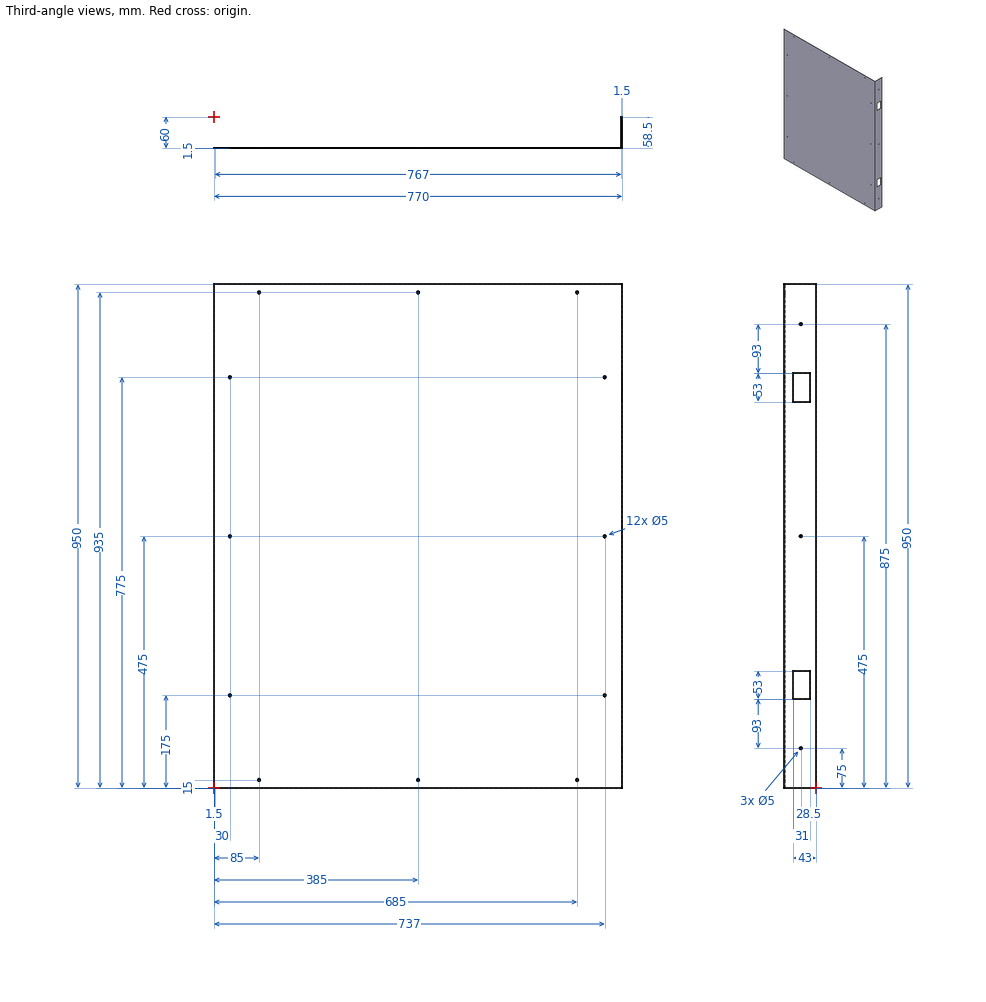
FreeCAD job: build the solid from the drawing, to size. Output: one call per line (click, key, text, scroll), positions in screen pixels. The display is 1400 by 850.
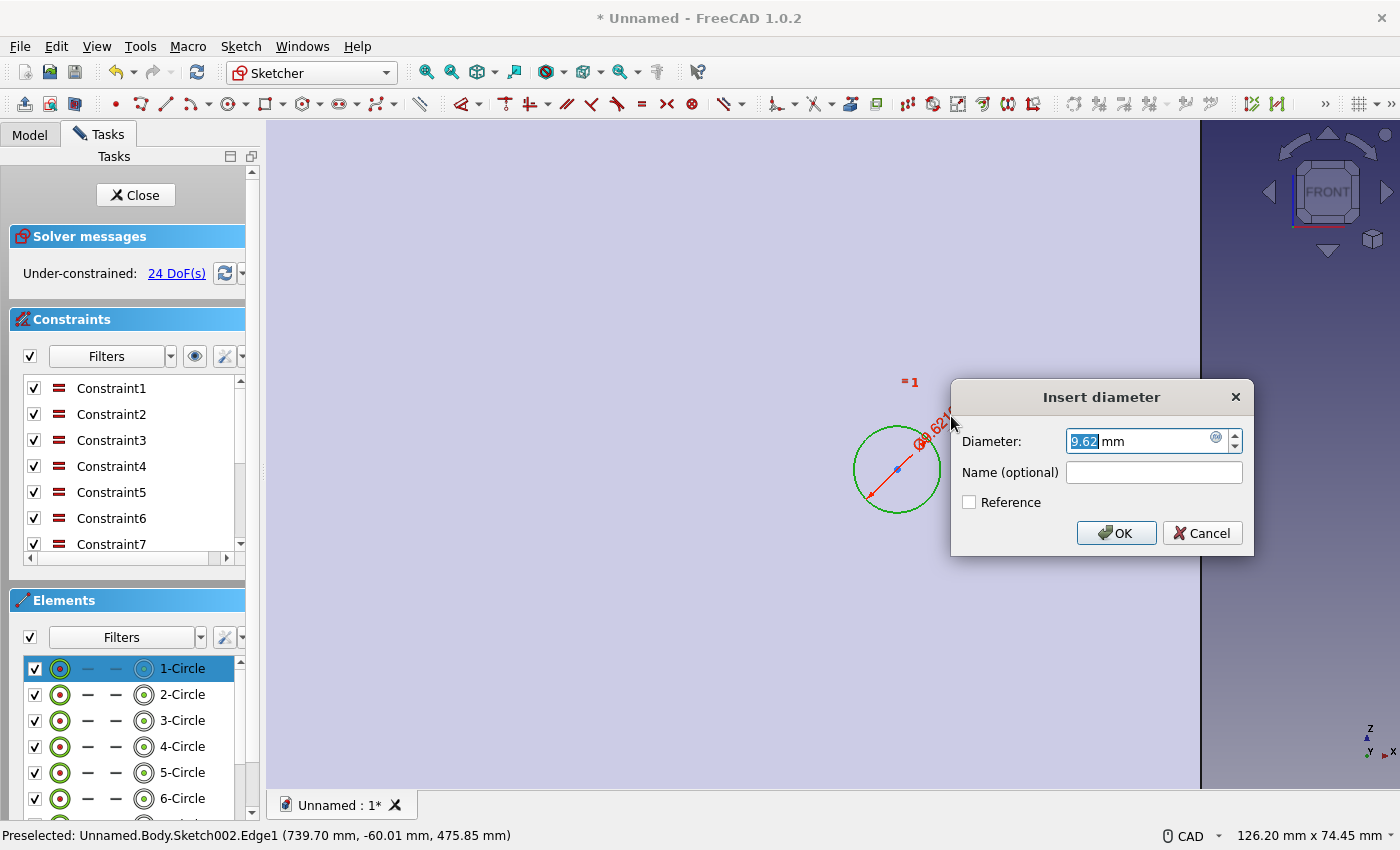
text(5)
key(Return)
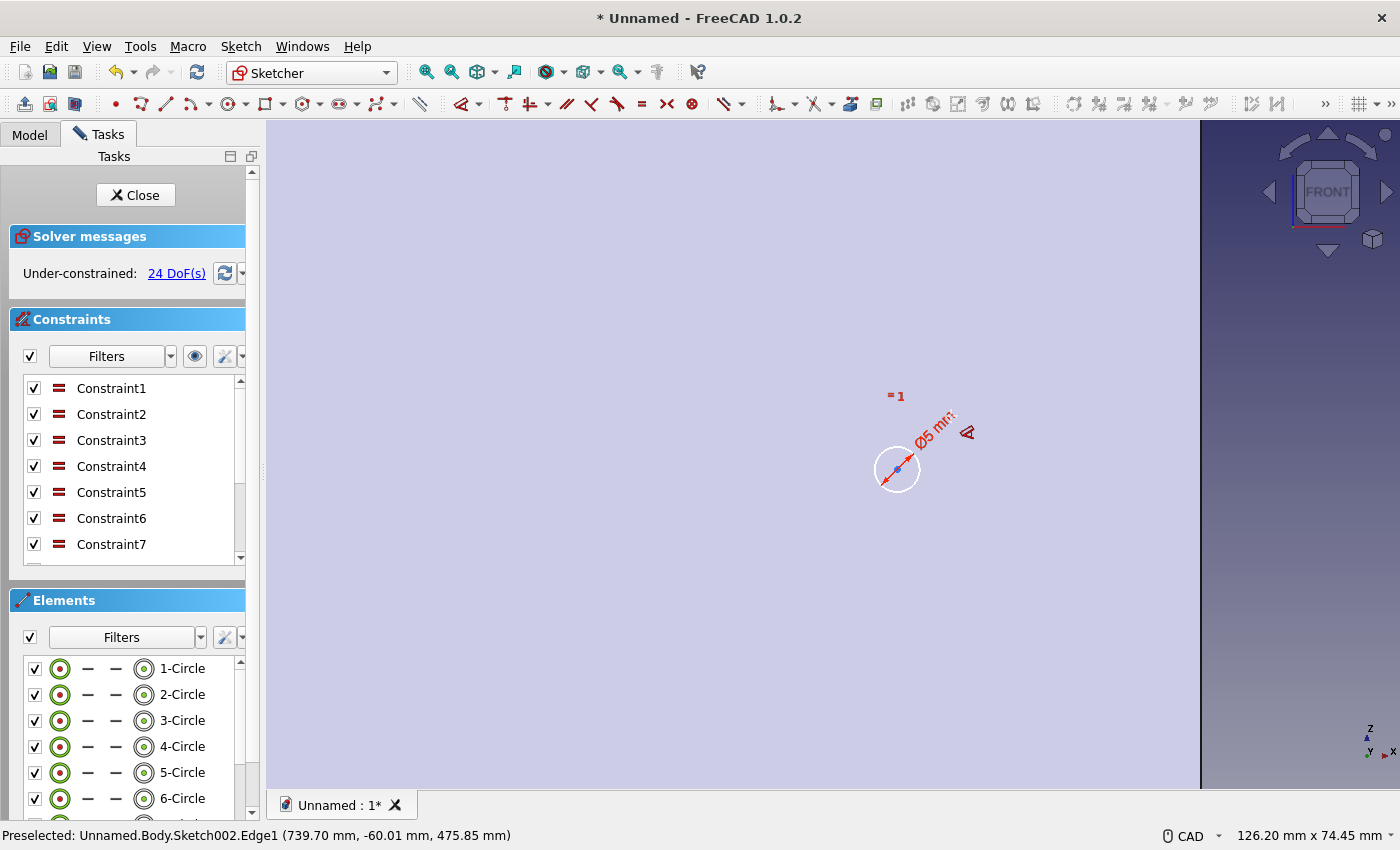
scroll(930, 452, down, 15)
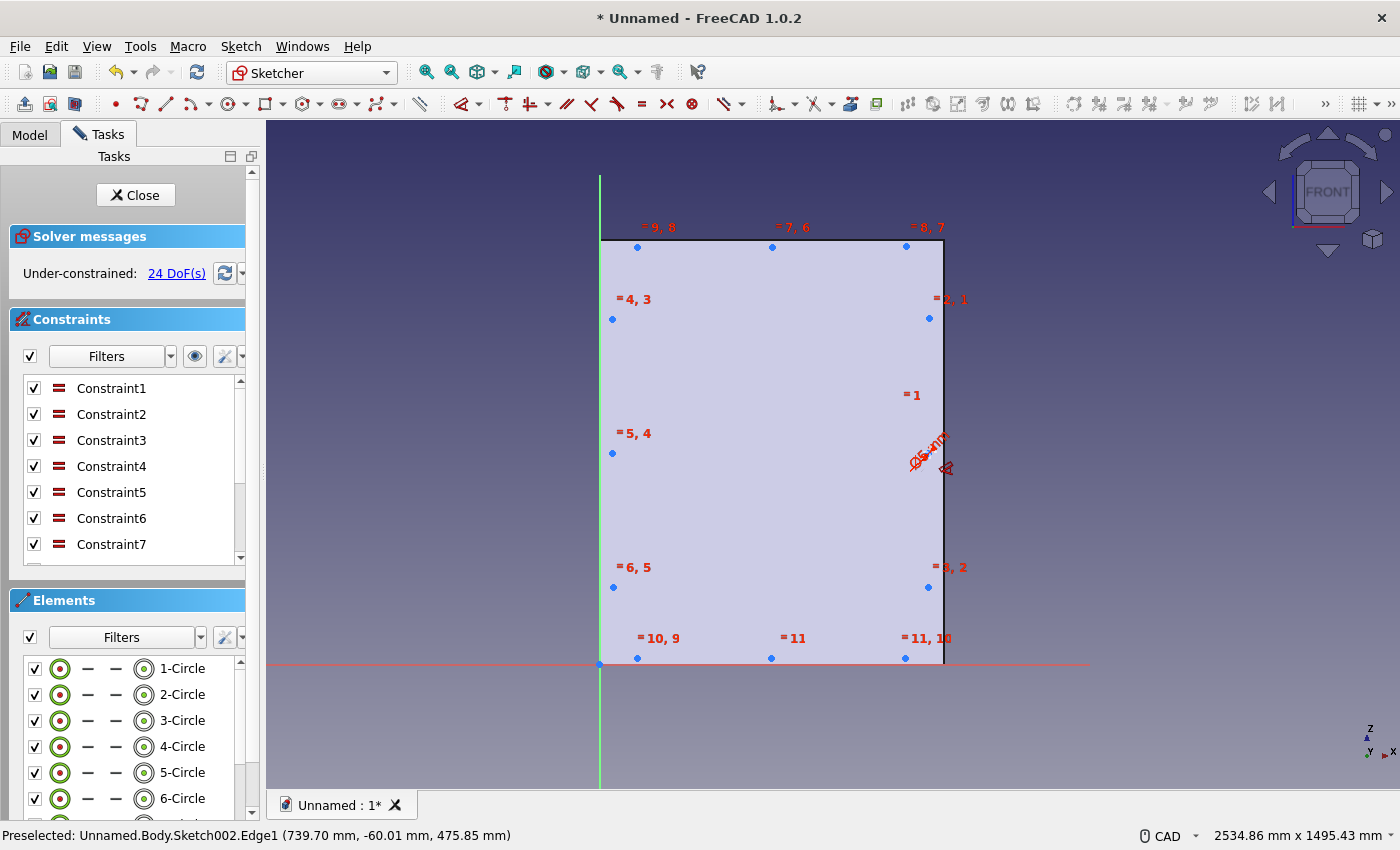
scroll(613, 319, up, 6)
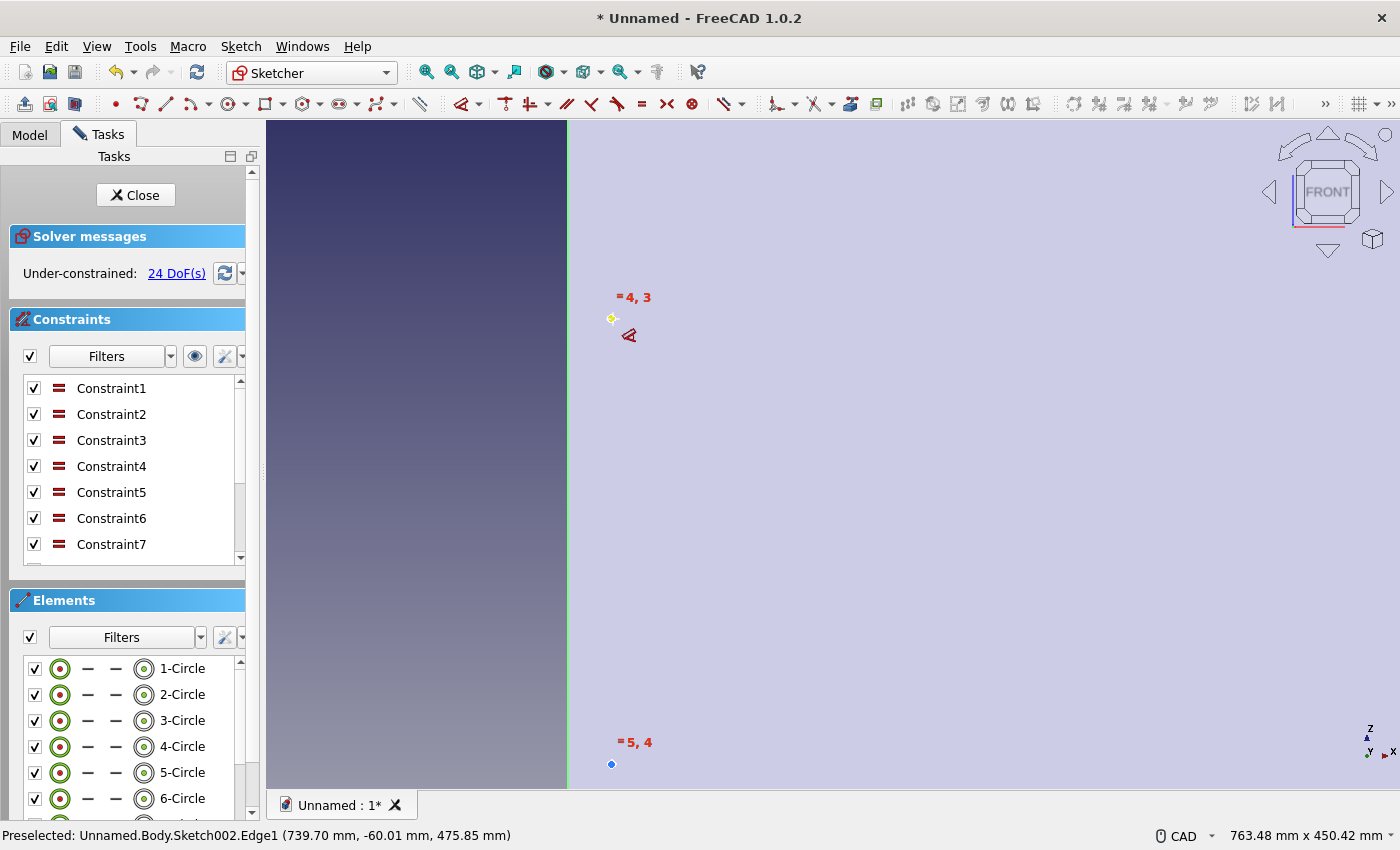
click(611, 319)
click(589, 285)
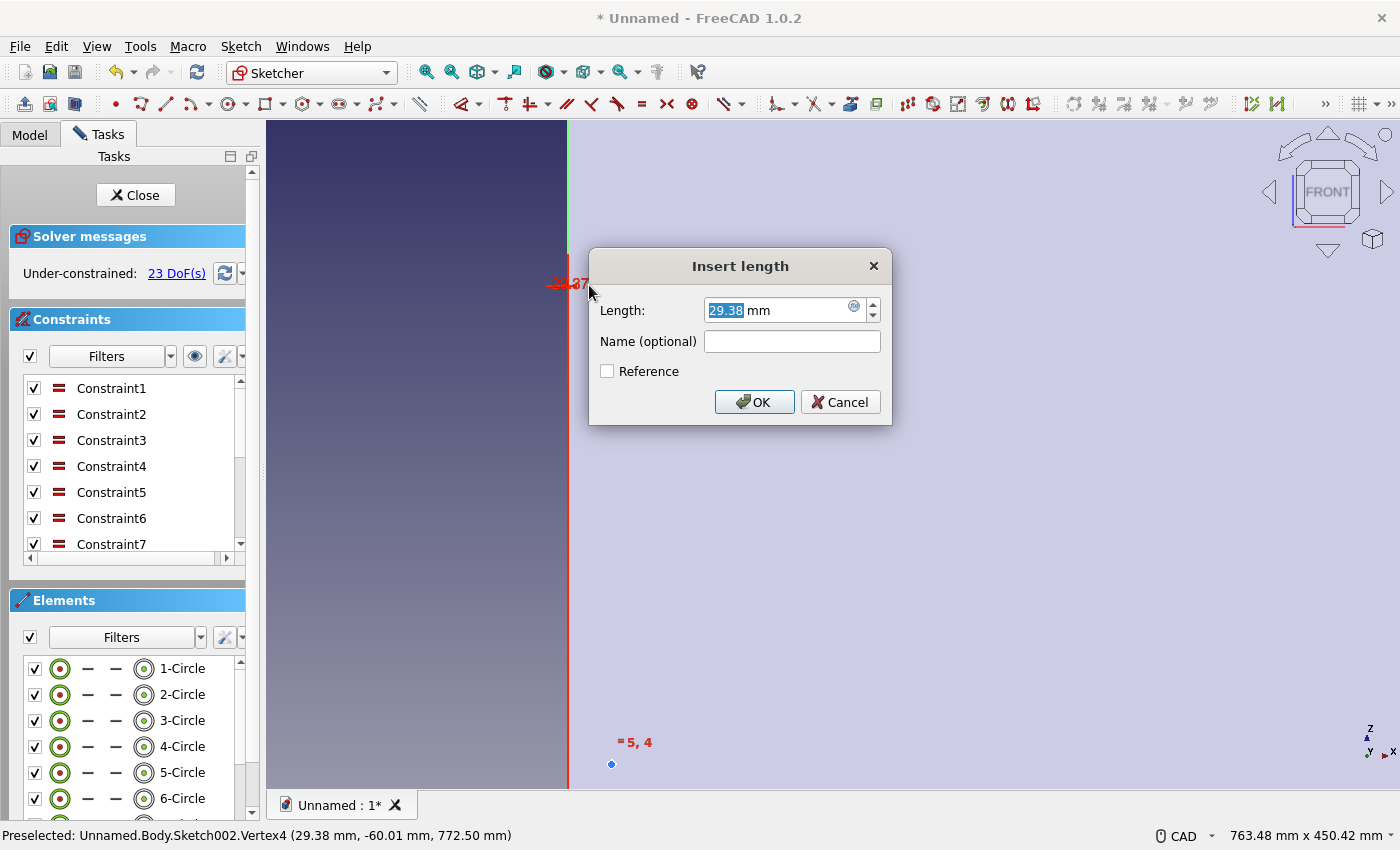
text(30)
key(Return)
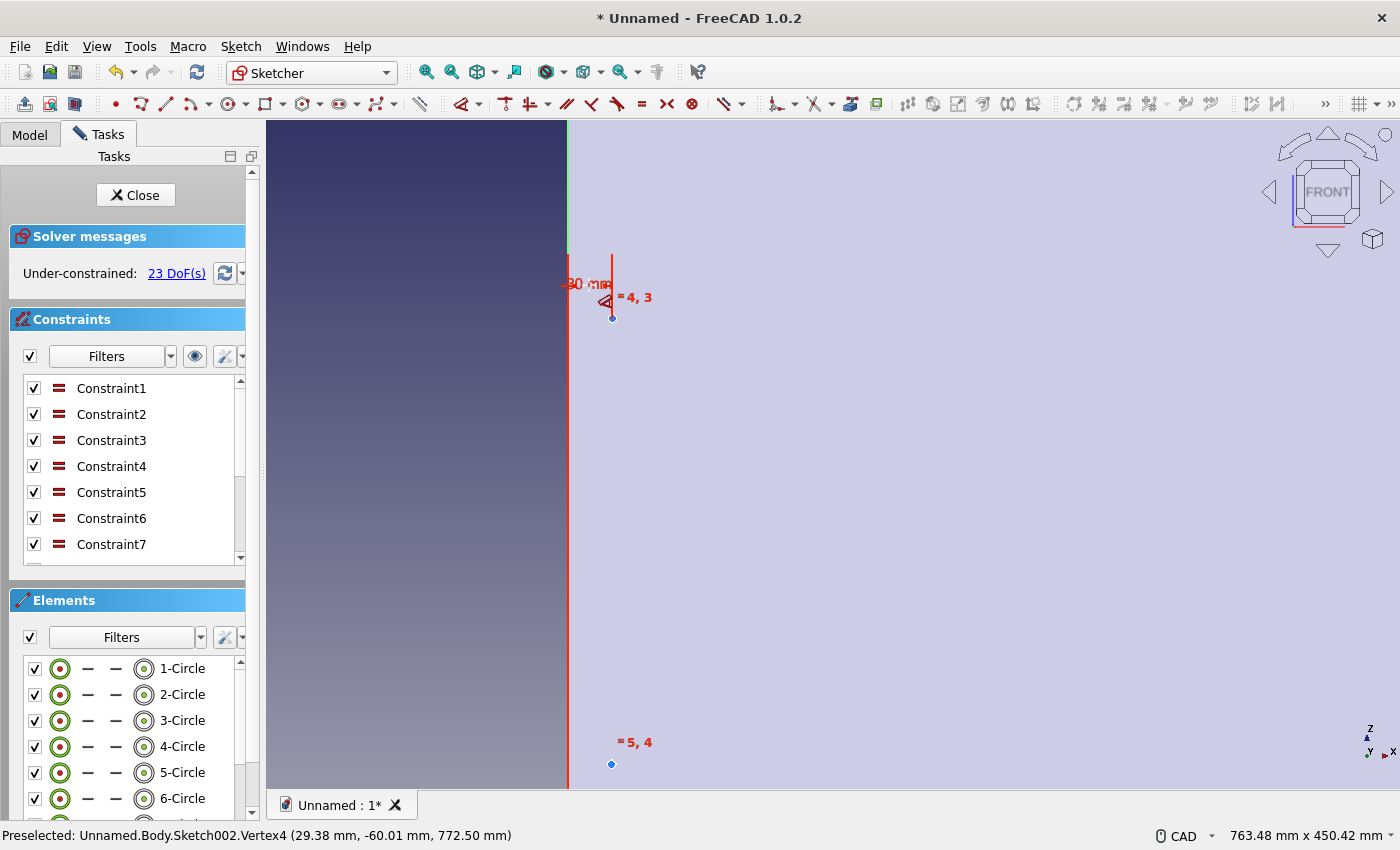
scroll(613, 319, down, 6)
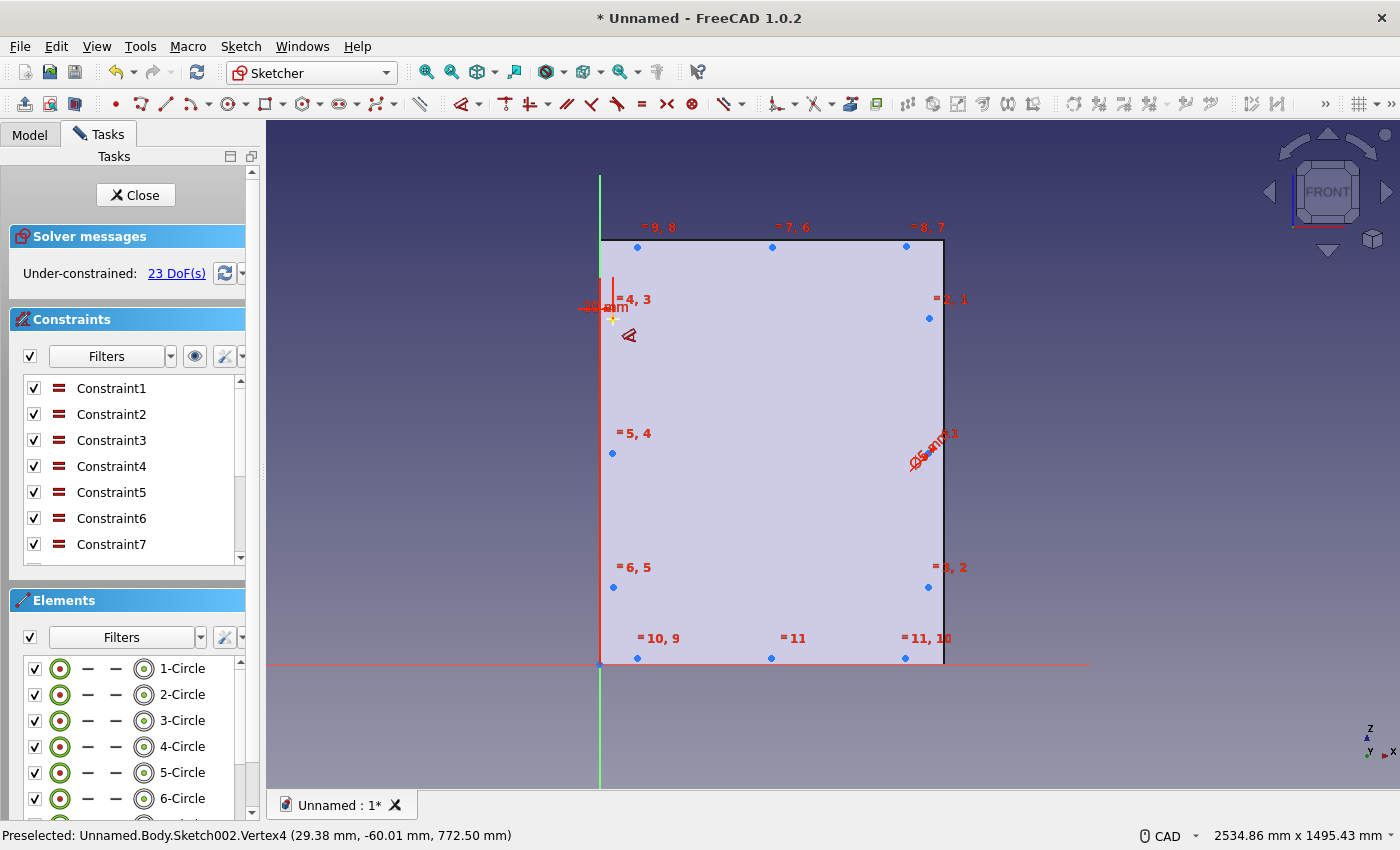
scroll(613, 453, up, 6)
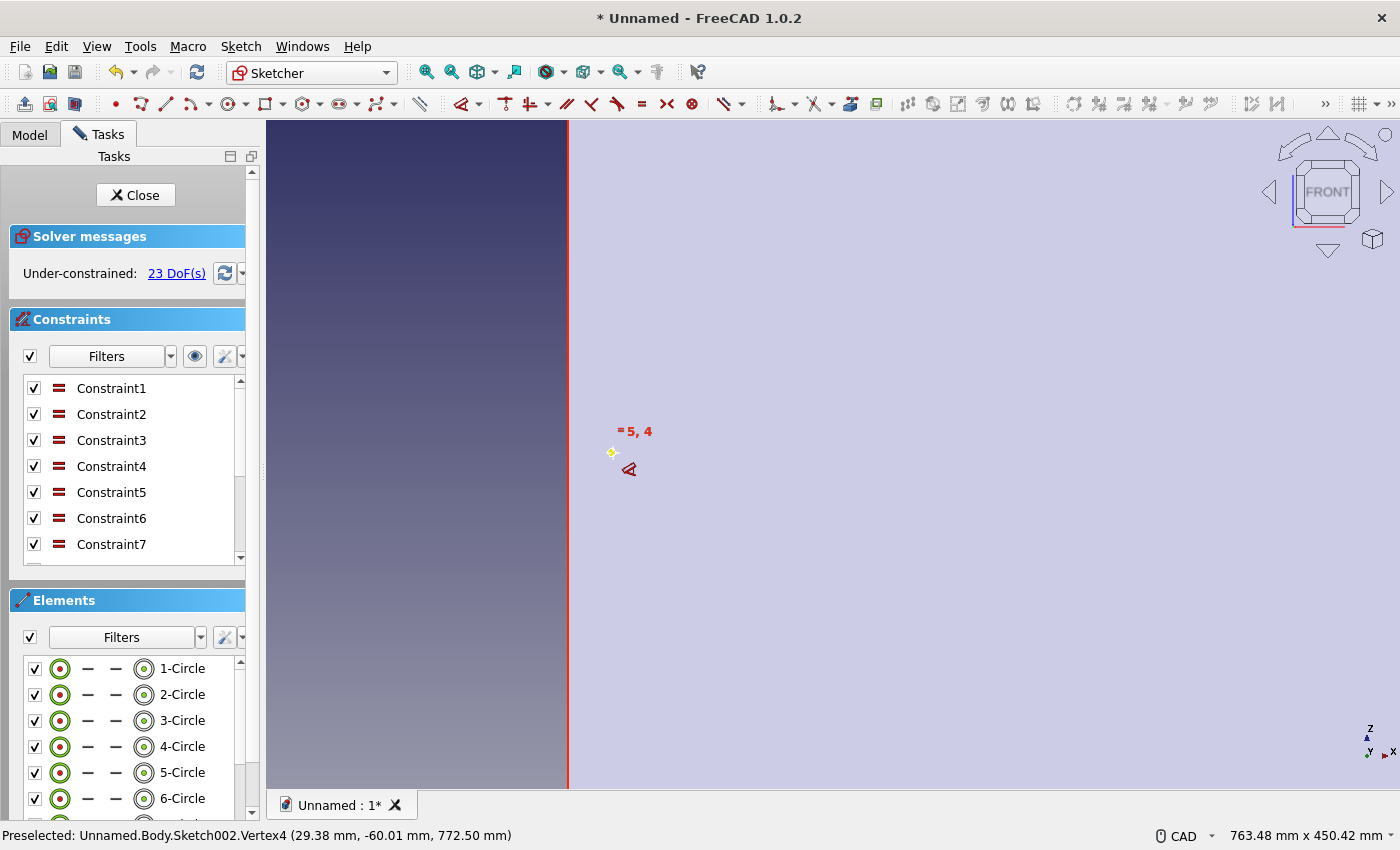
click(612, 453)
click(590, 419)